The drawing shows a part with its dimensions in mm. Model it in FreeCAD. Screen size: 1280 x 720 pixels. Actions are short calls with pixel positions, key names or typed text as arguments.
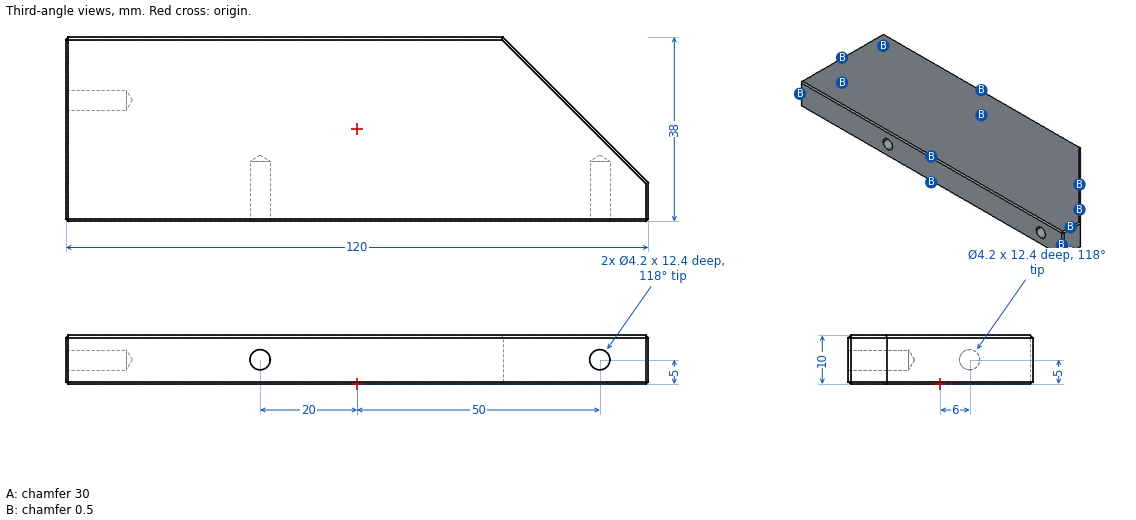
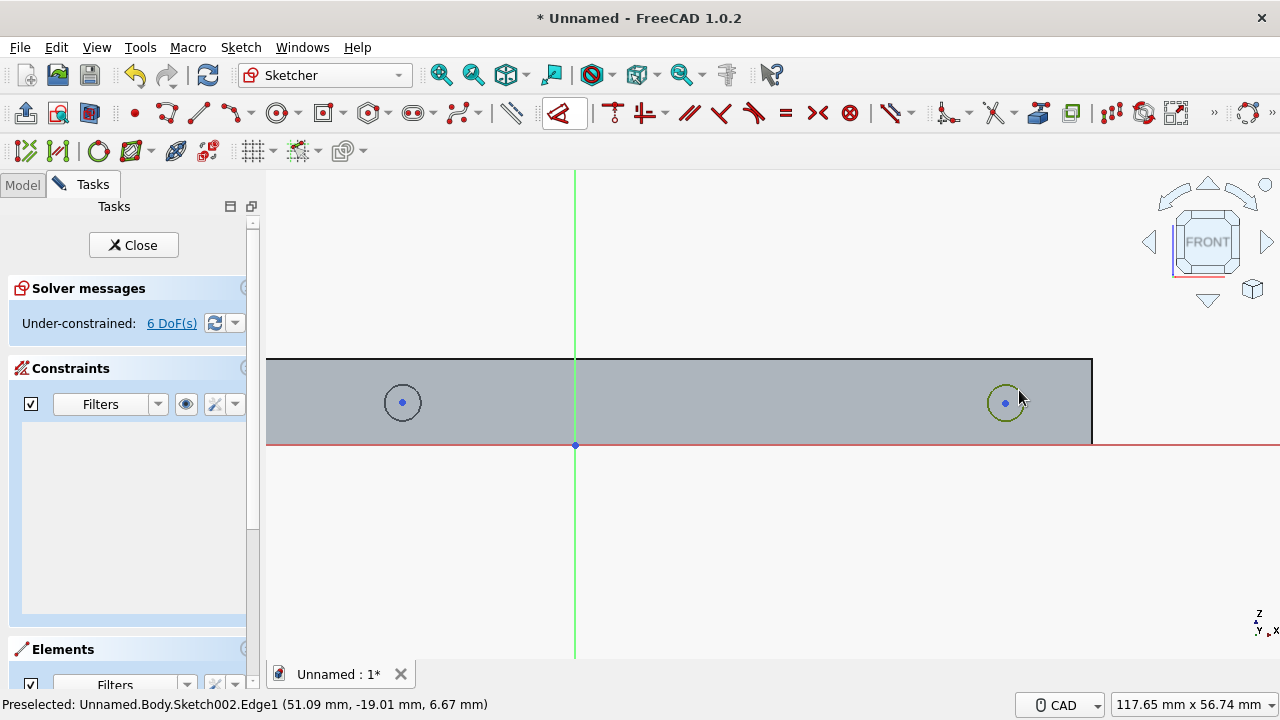
click(415, 390)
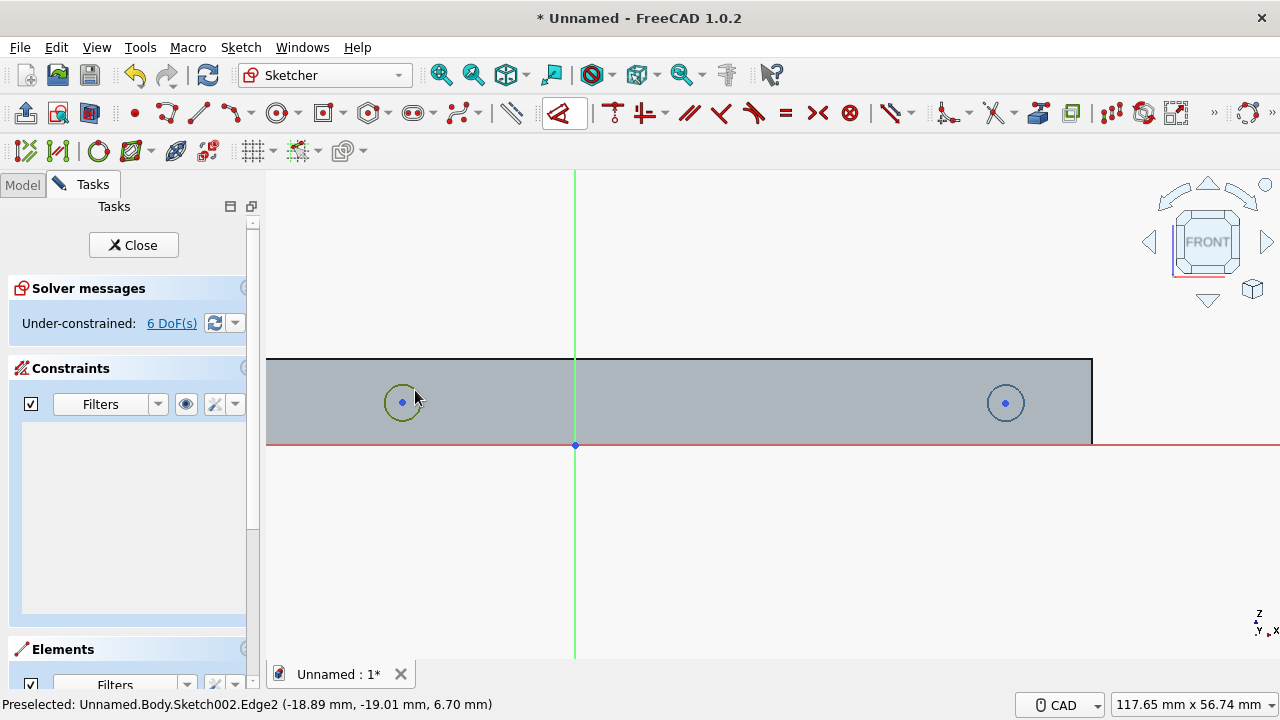
click(786, 114)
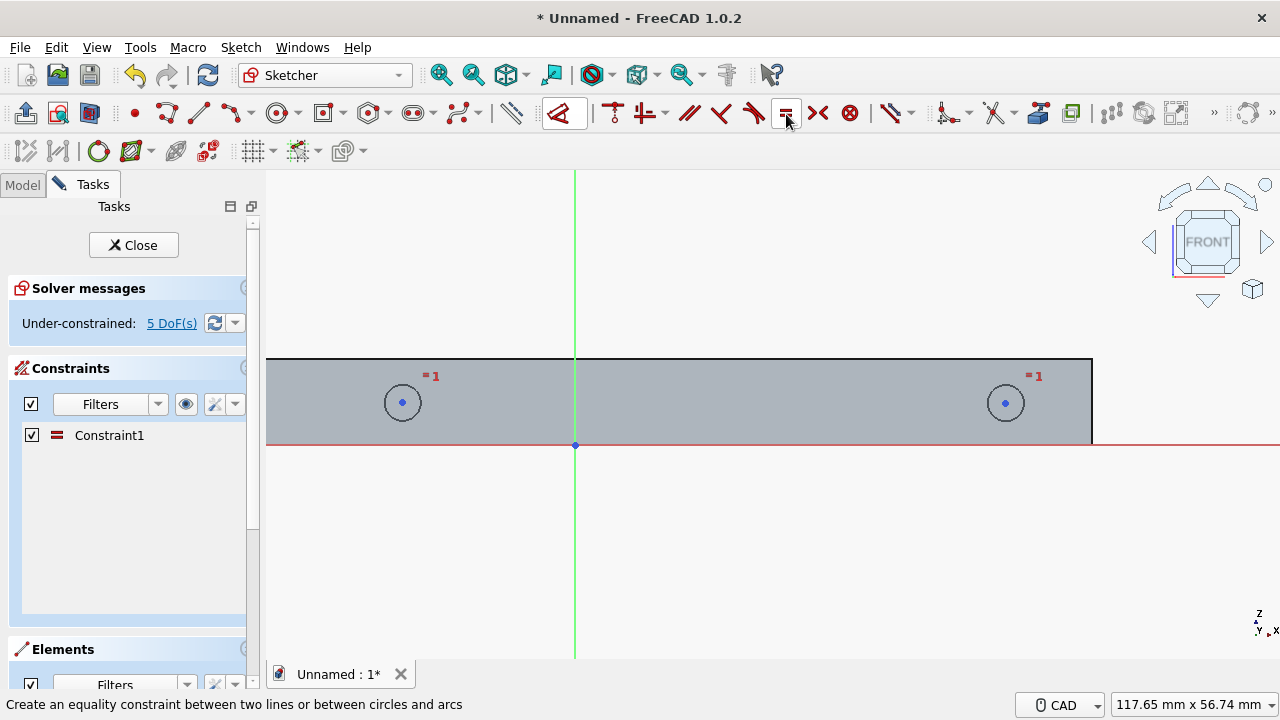
click(1019, 390)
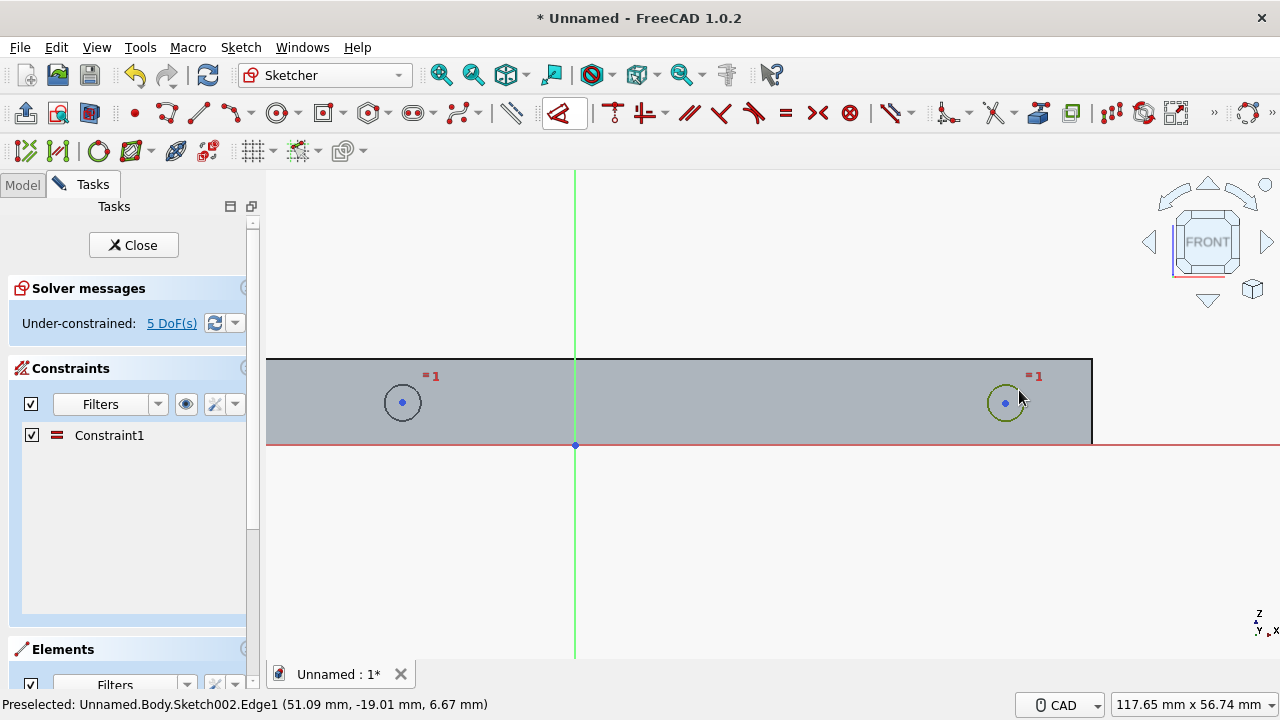
click(582, 114)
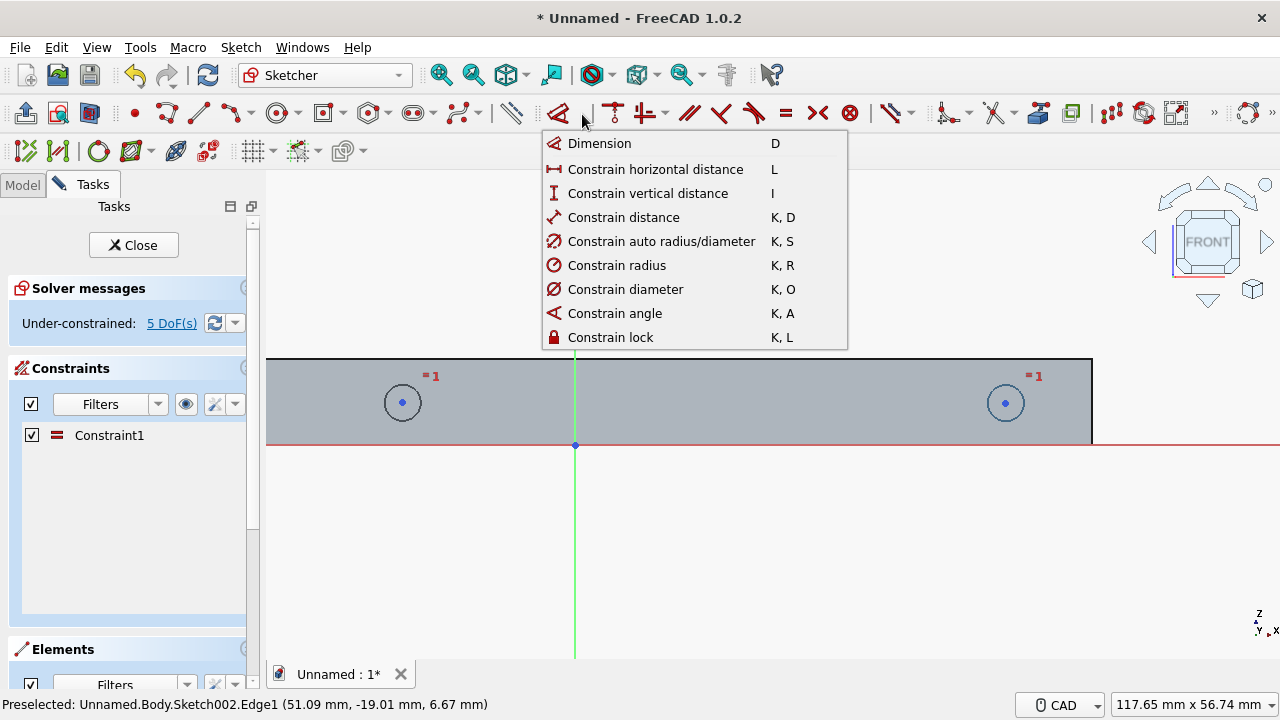
click(695, 289)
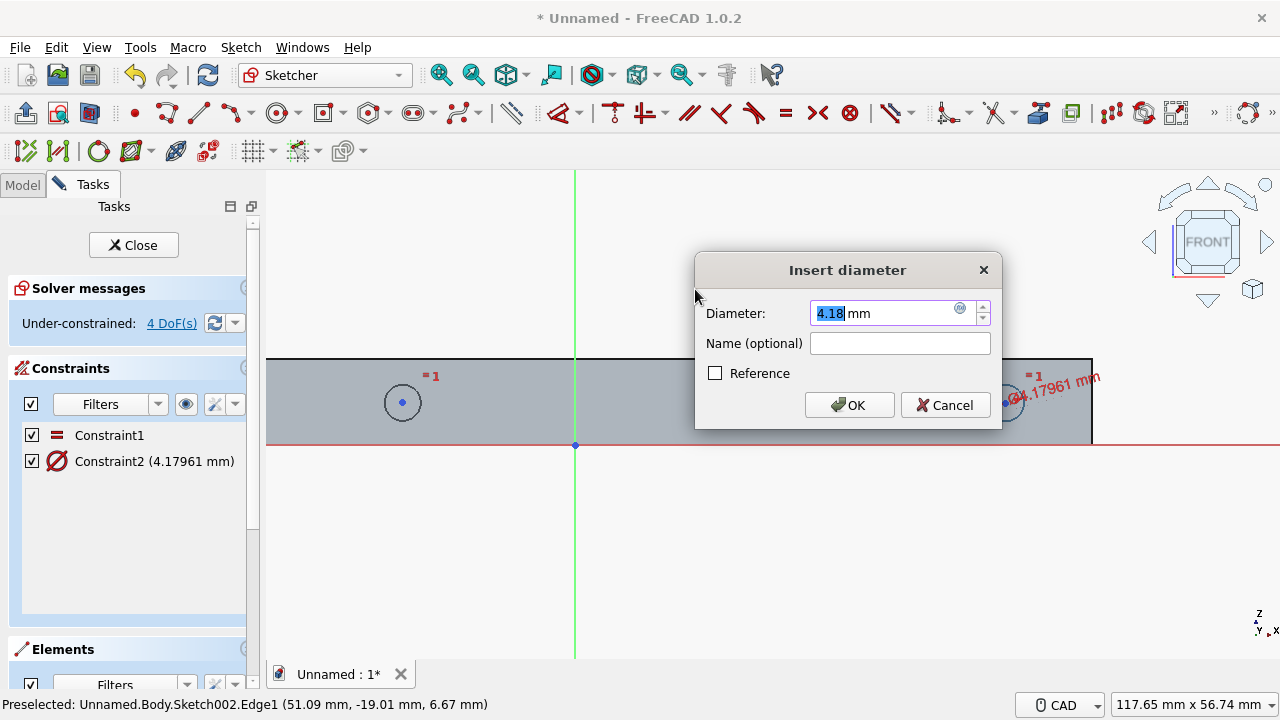
text(4.2)
key(Return)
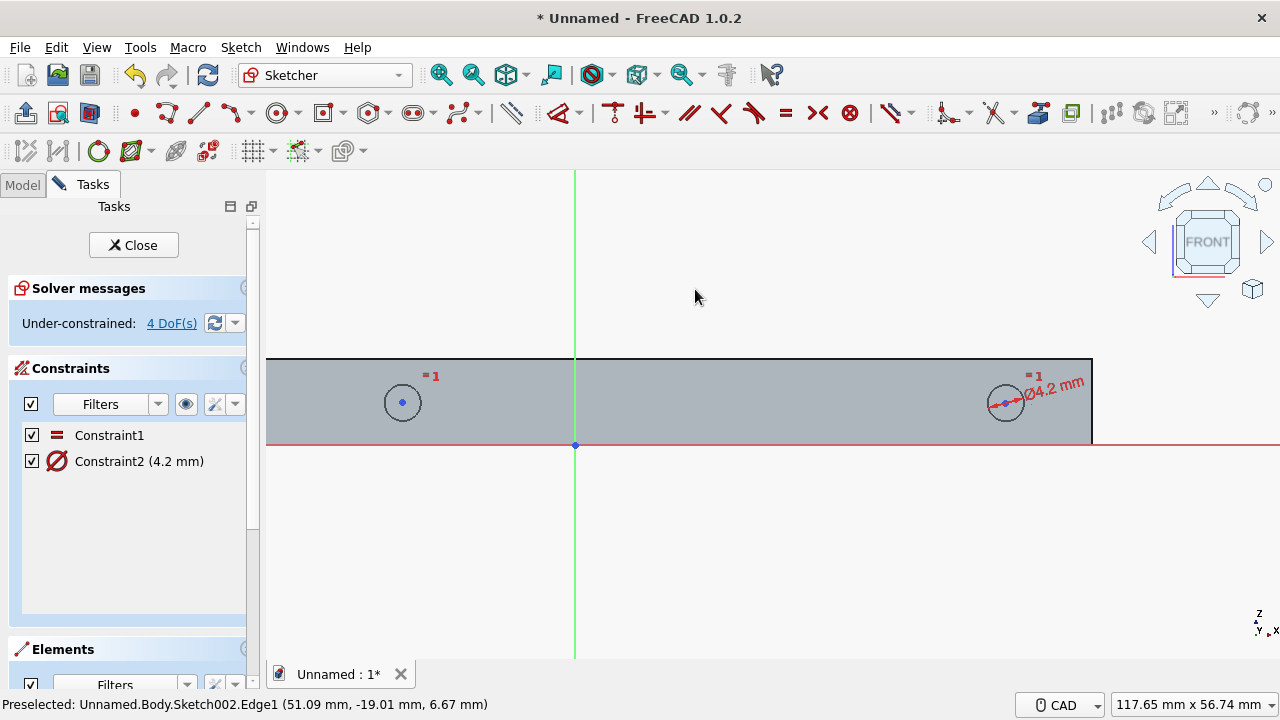
click(1006, 403)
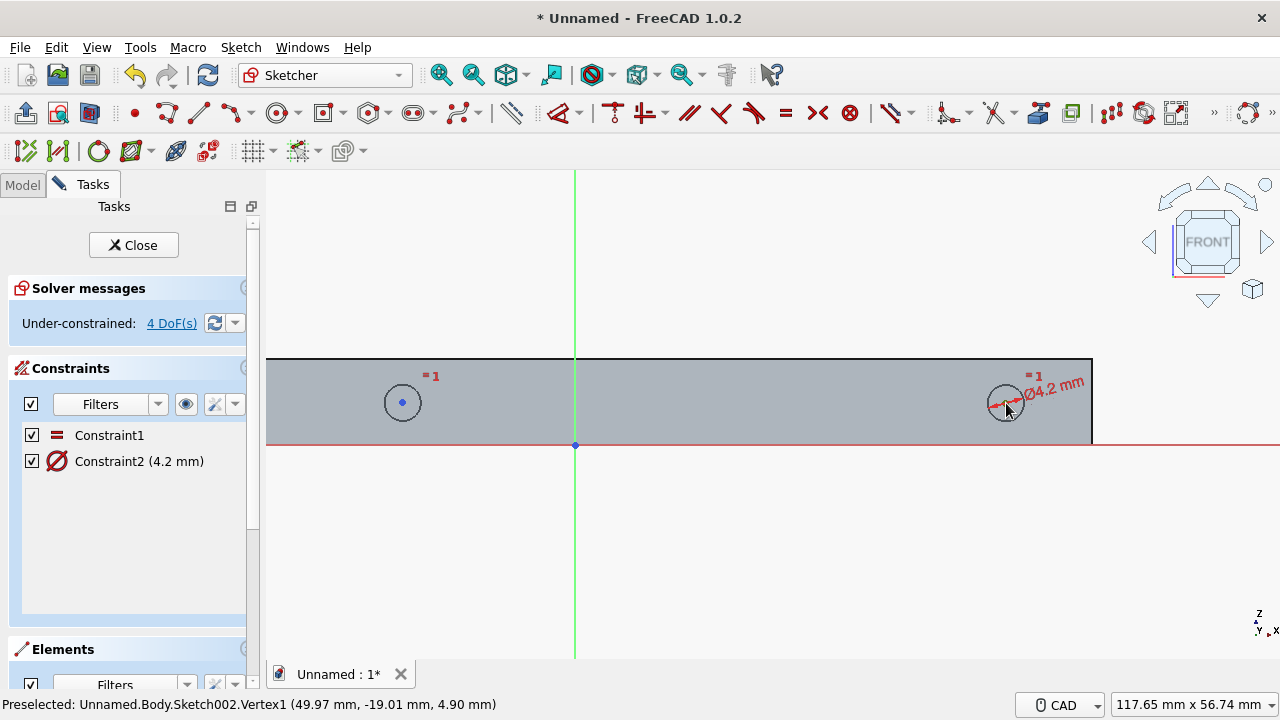
key(i)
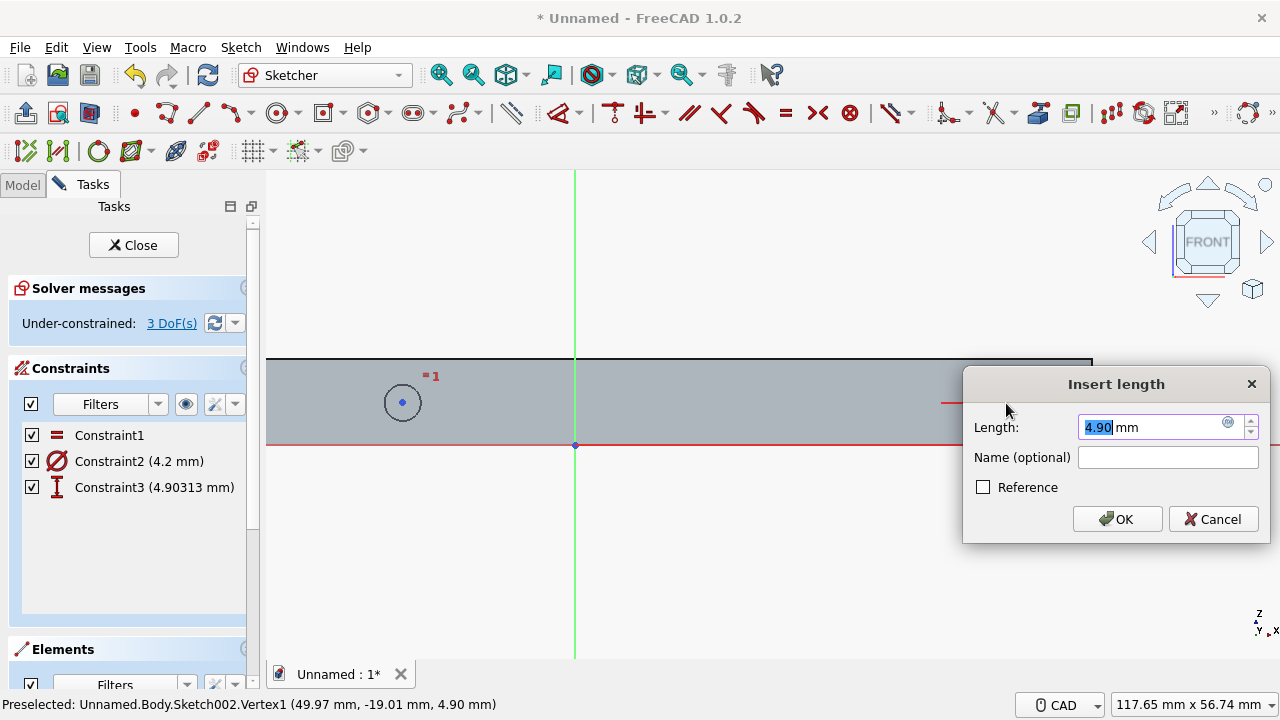
text(5)
key(Return)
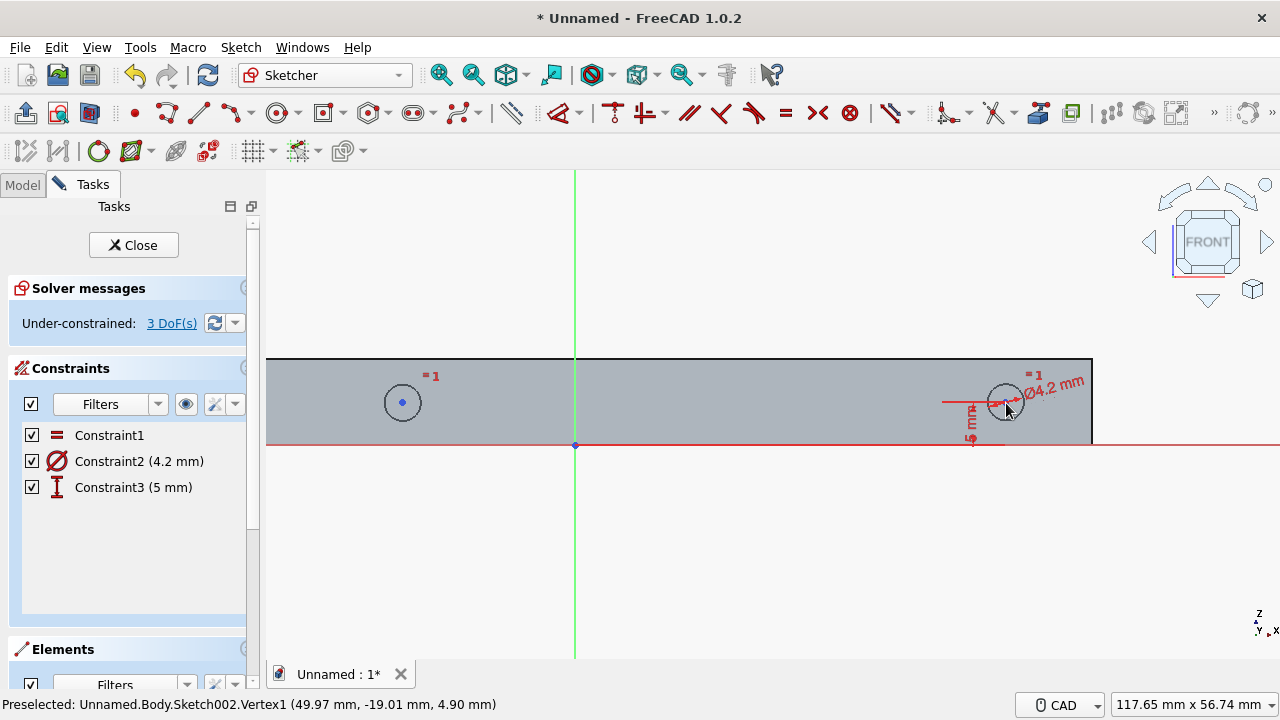
click(403, 403)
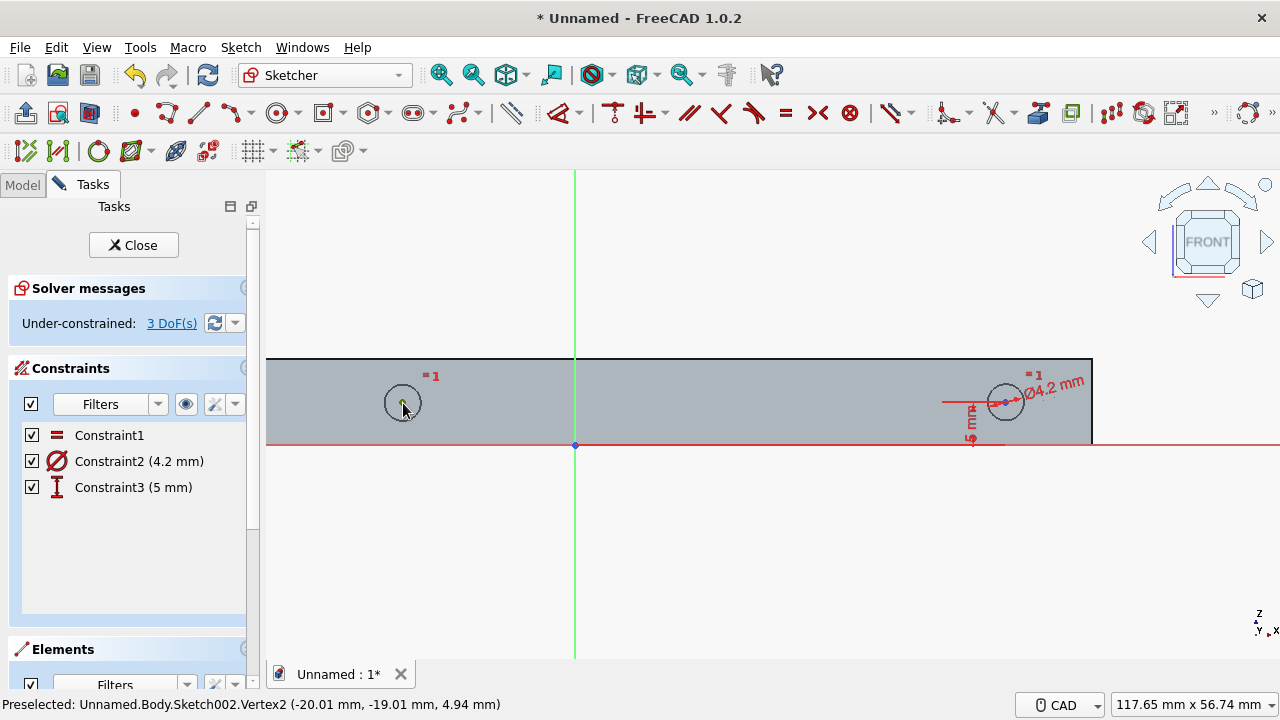
click(582, 114)